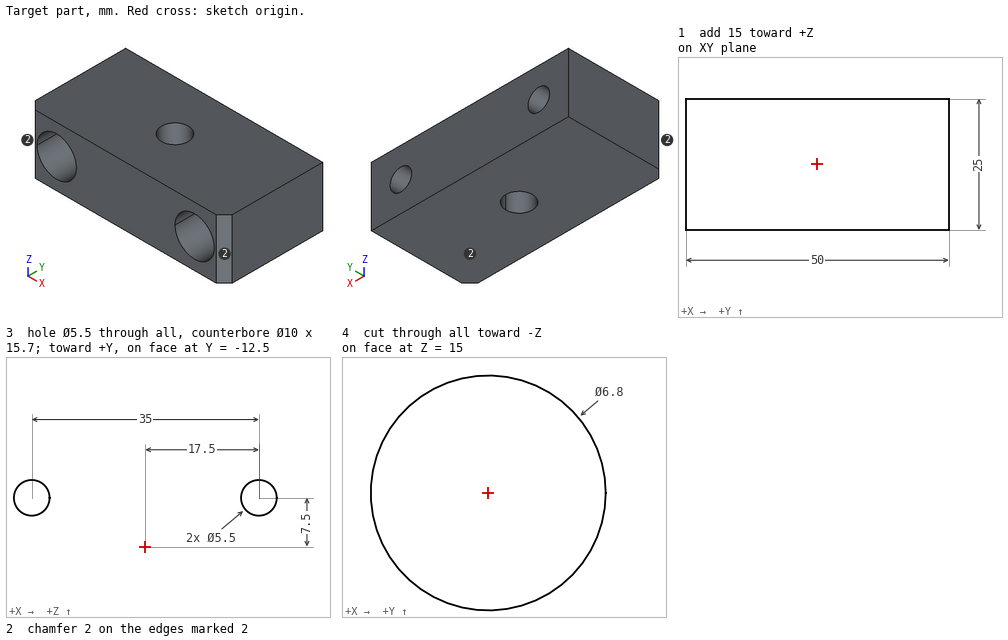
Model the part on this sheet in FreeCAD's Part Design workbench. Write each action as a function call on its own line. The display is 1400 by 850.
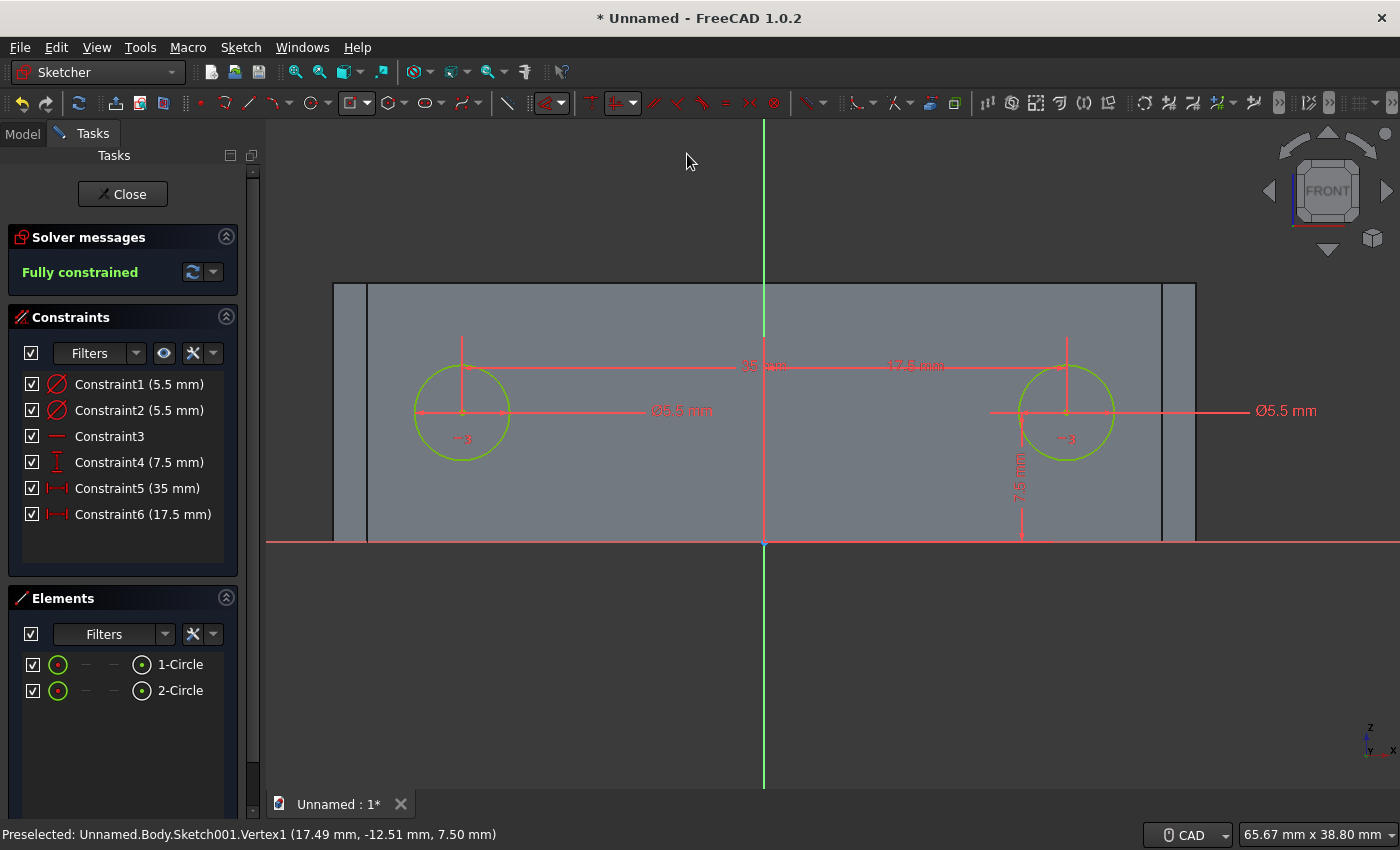
click(123, 194)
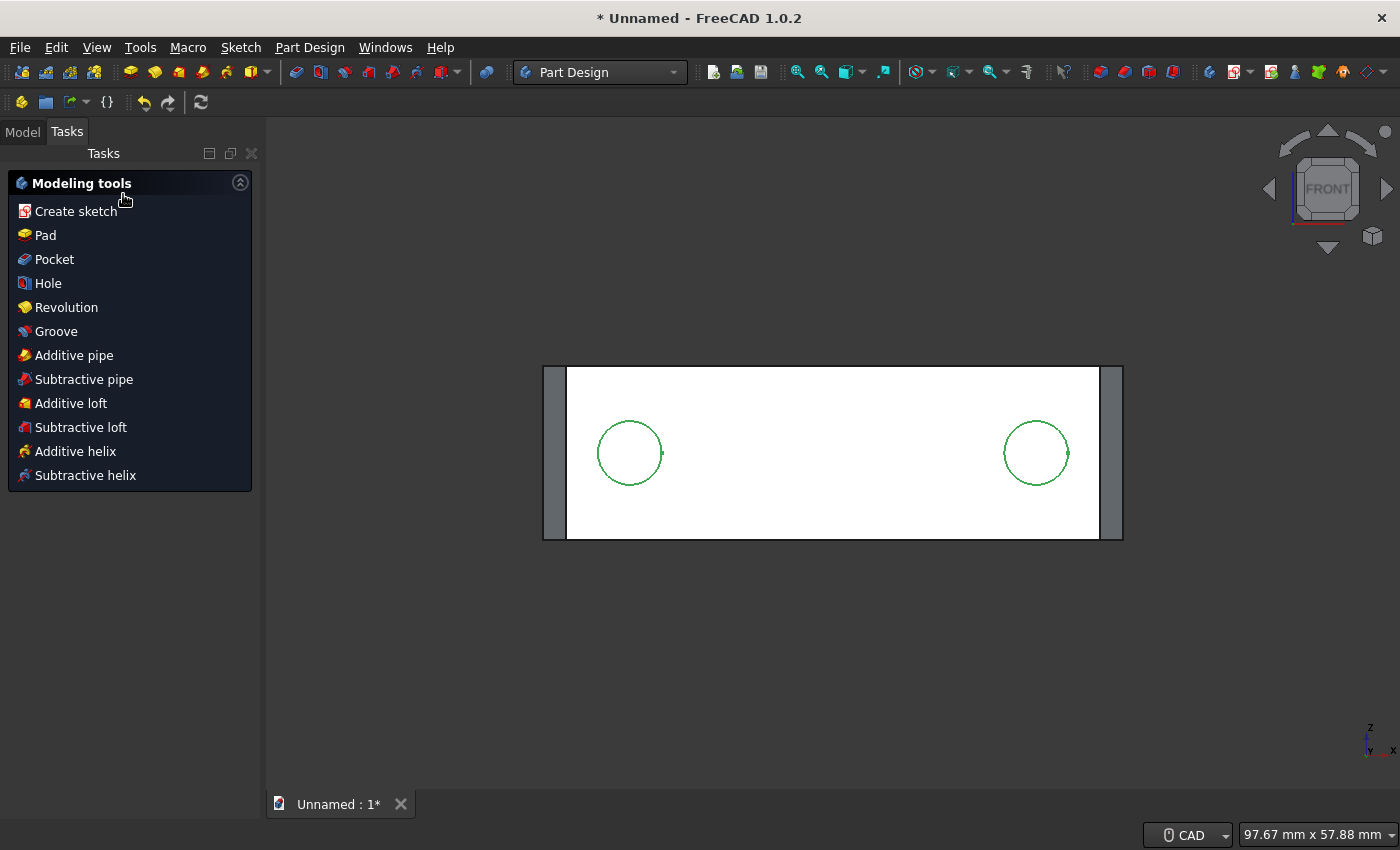
click(322, 72)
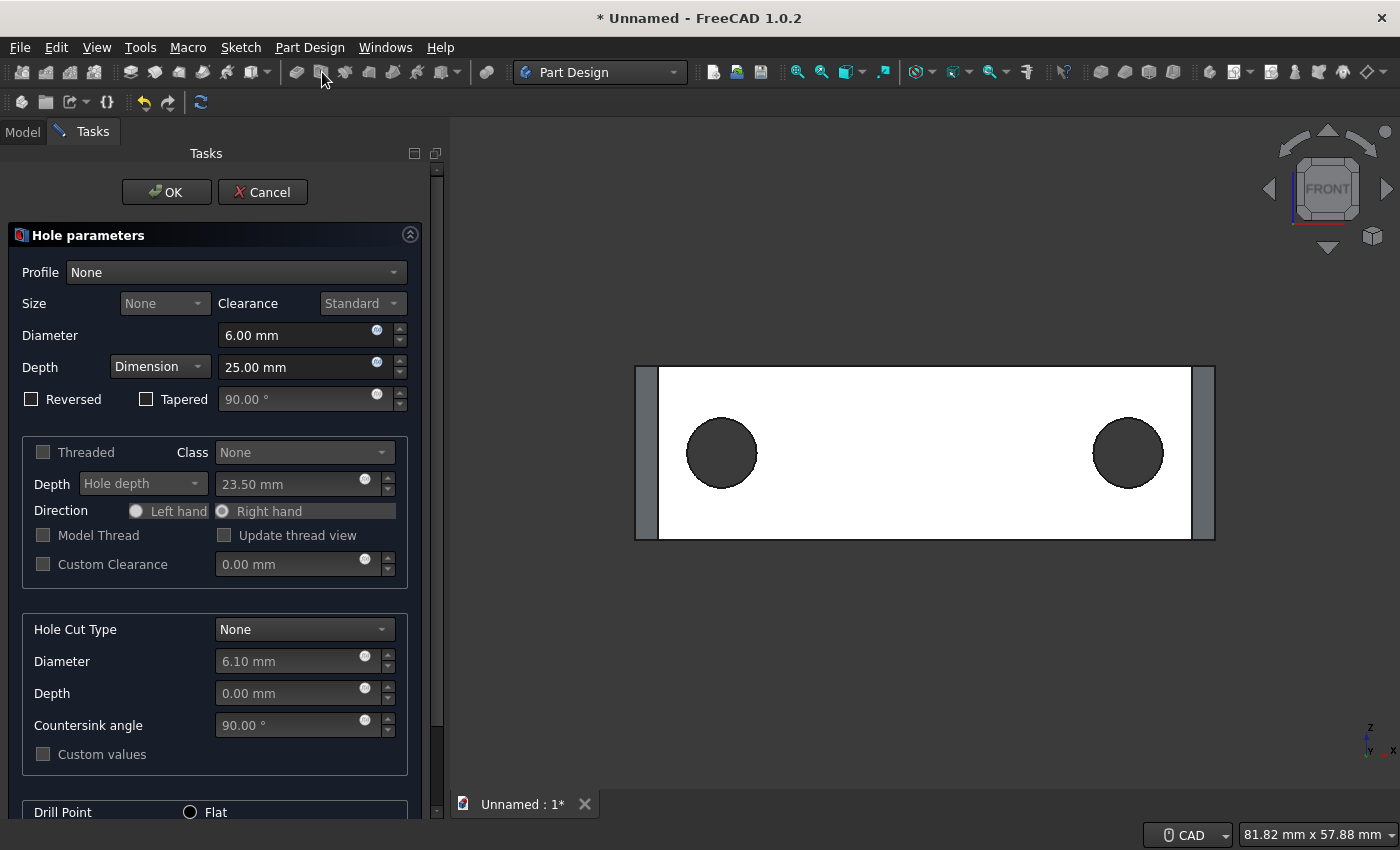
triple_click(305, 335)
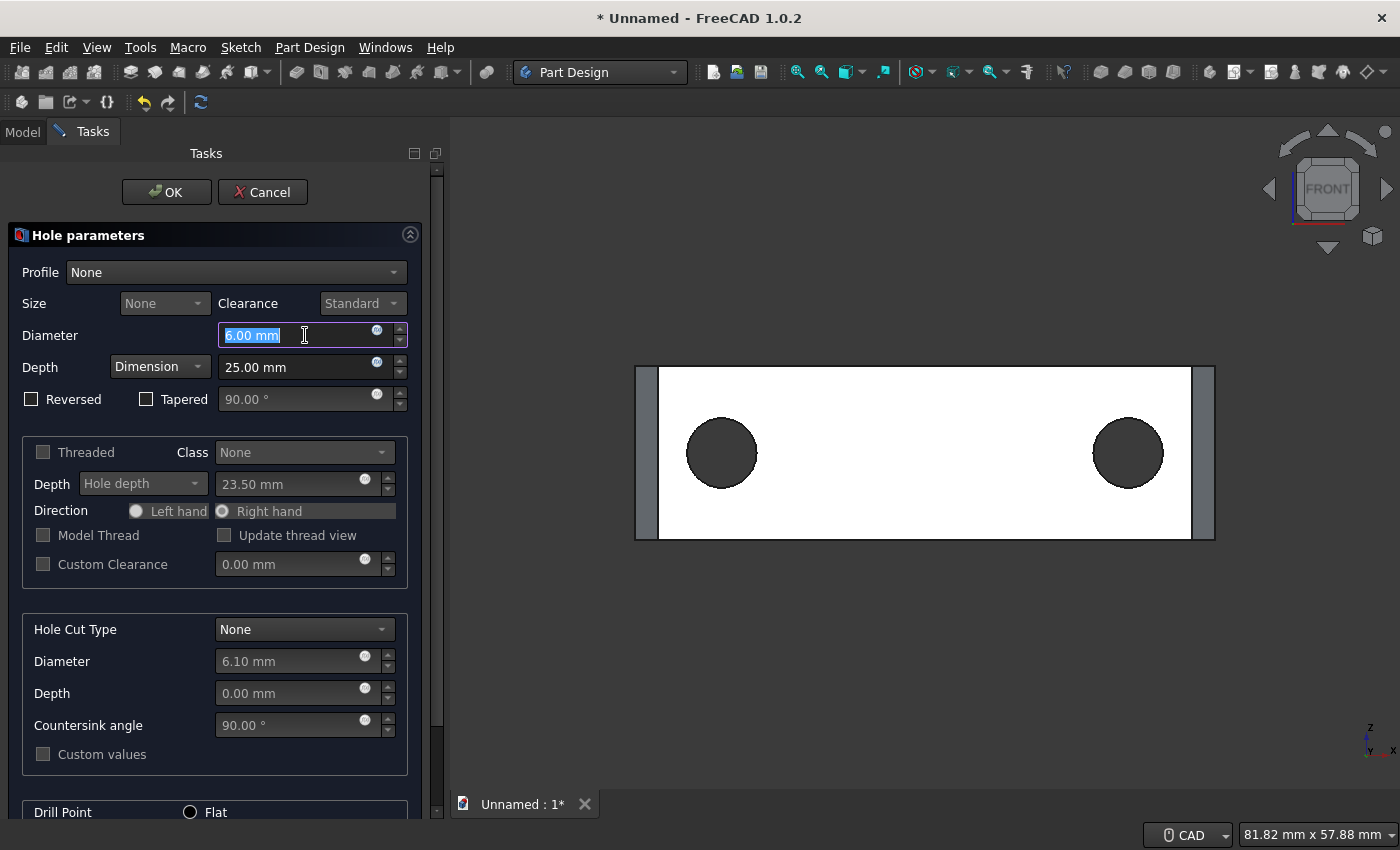
text(5.5)
key(Tab)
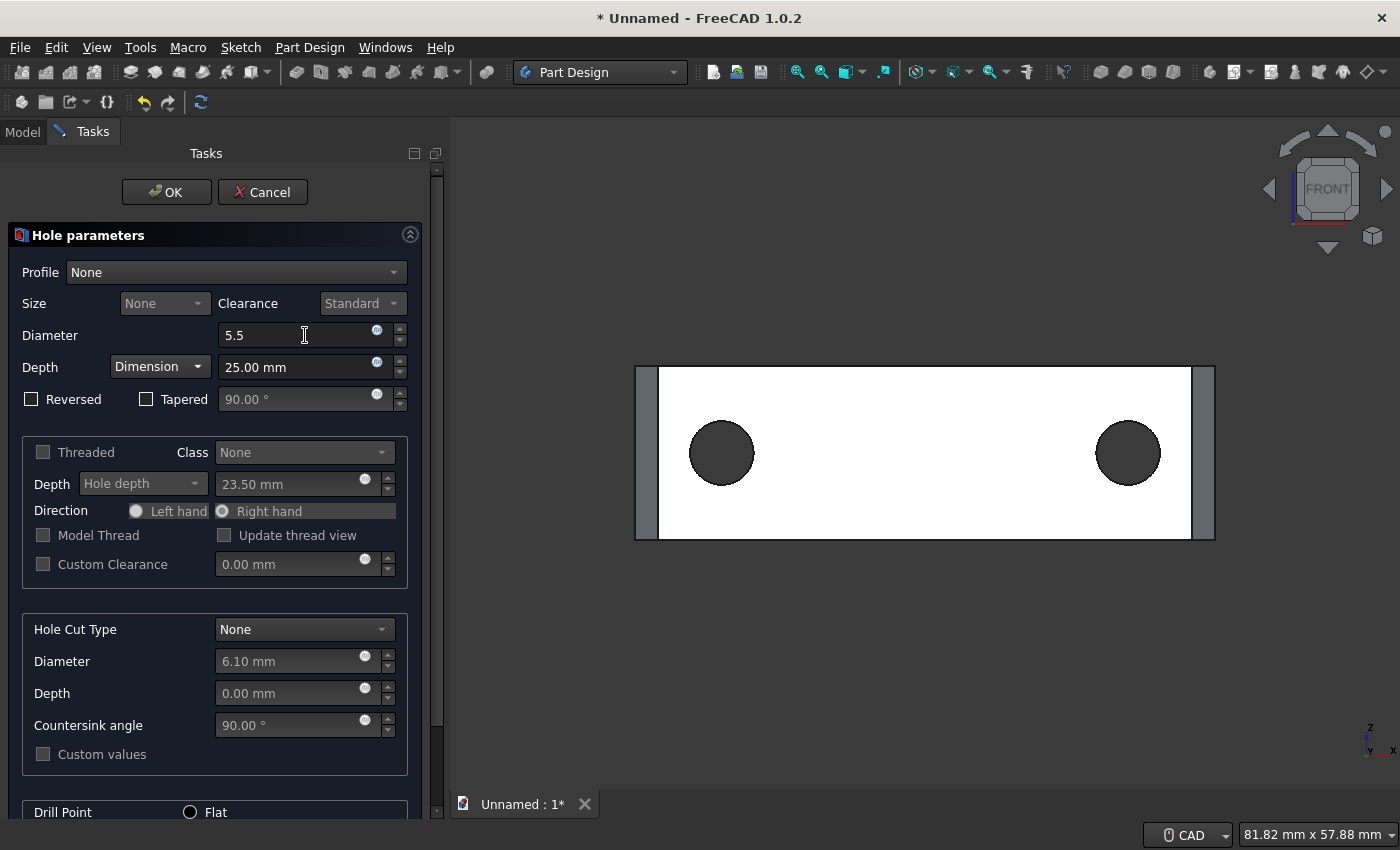
click(161, 366)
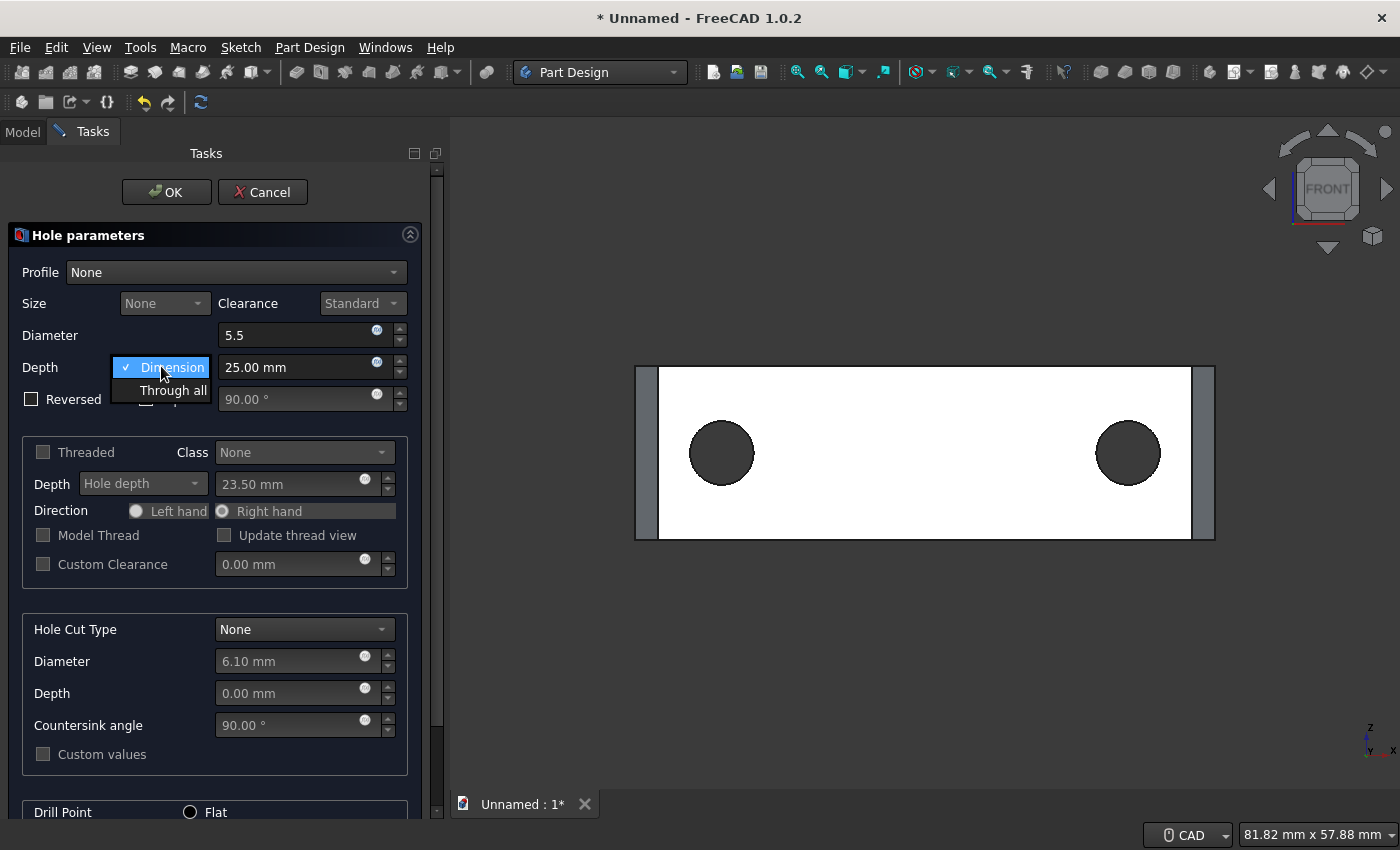
click(160, 390)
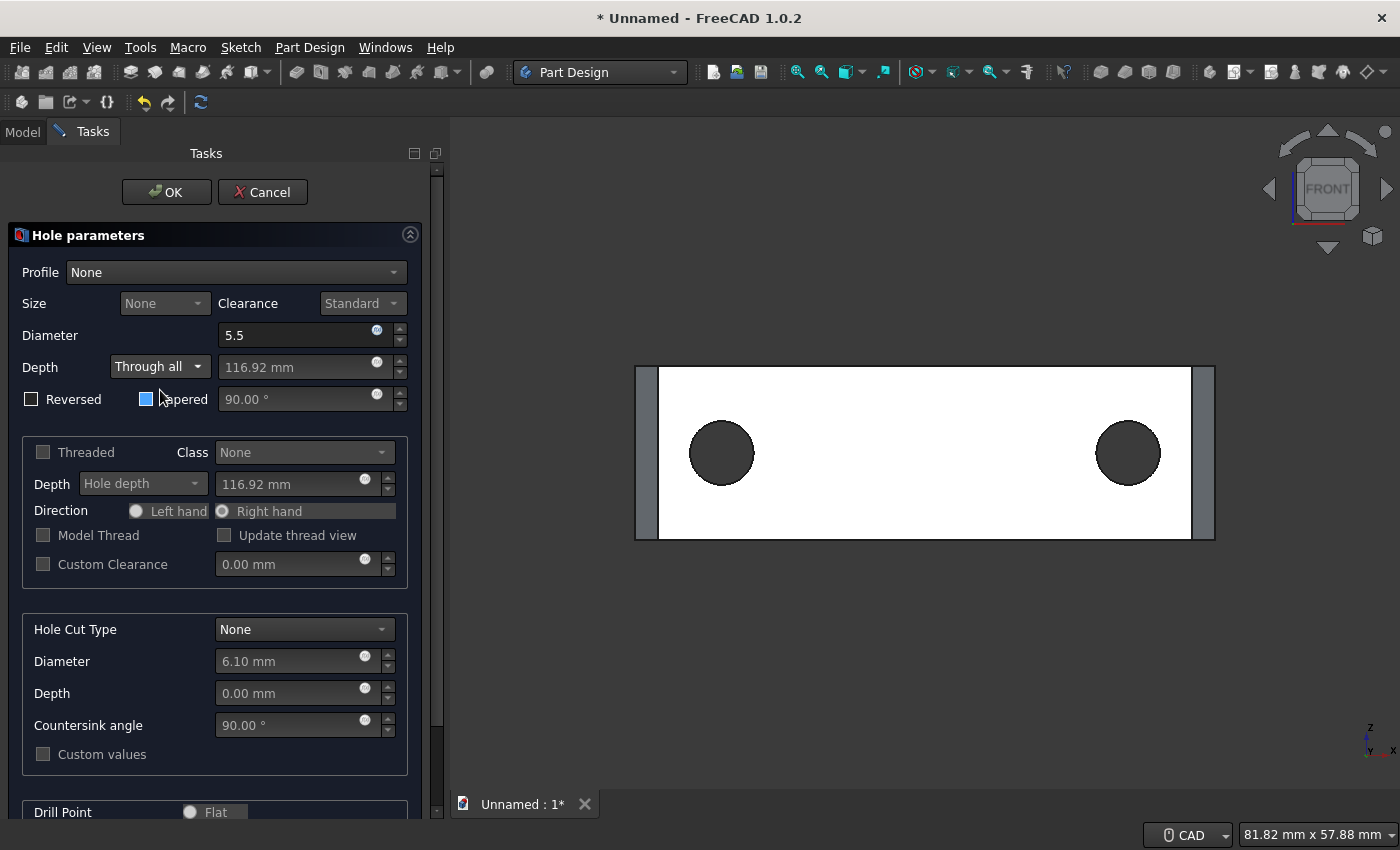
click(306, 630)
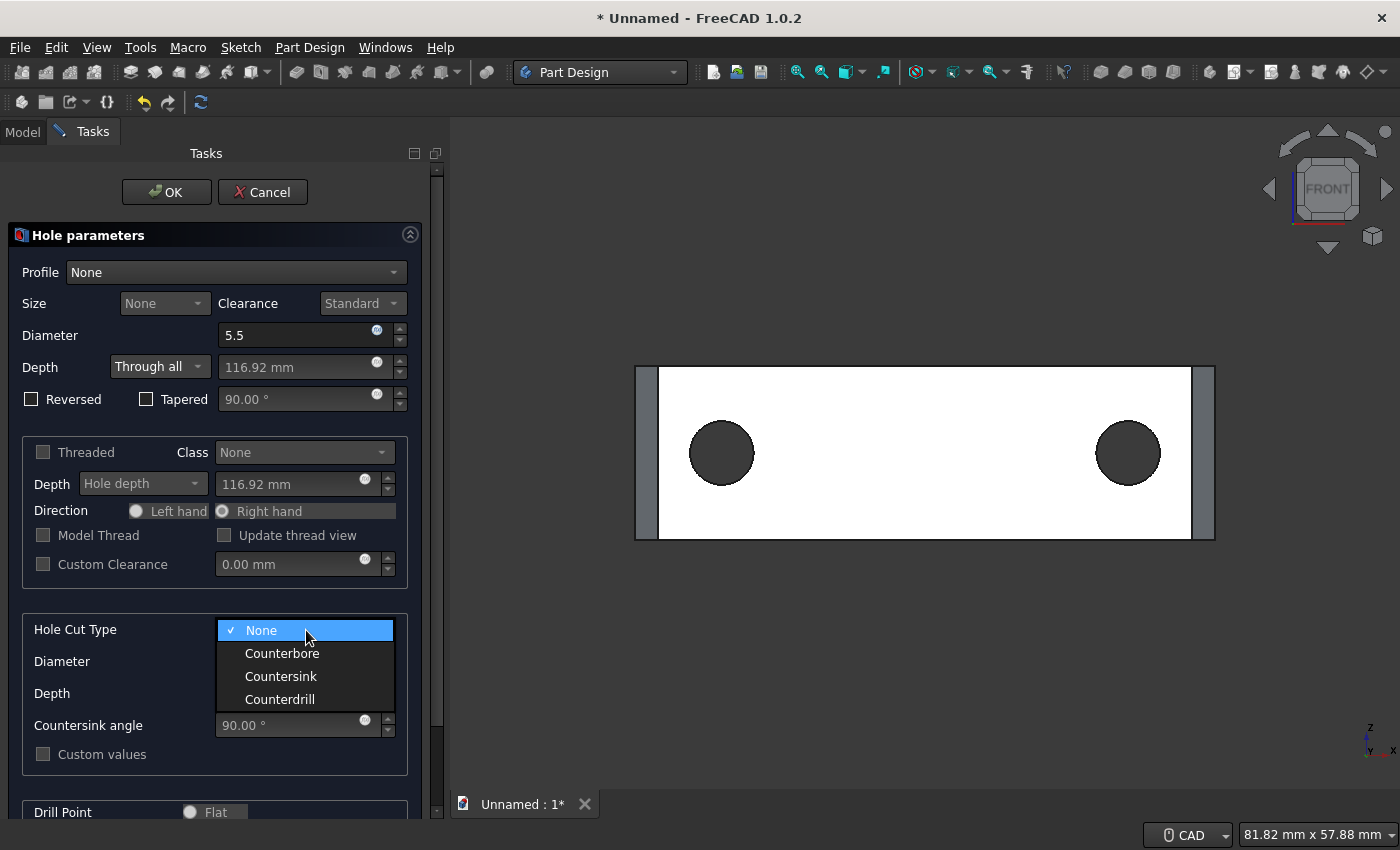
click(304, 654)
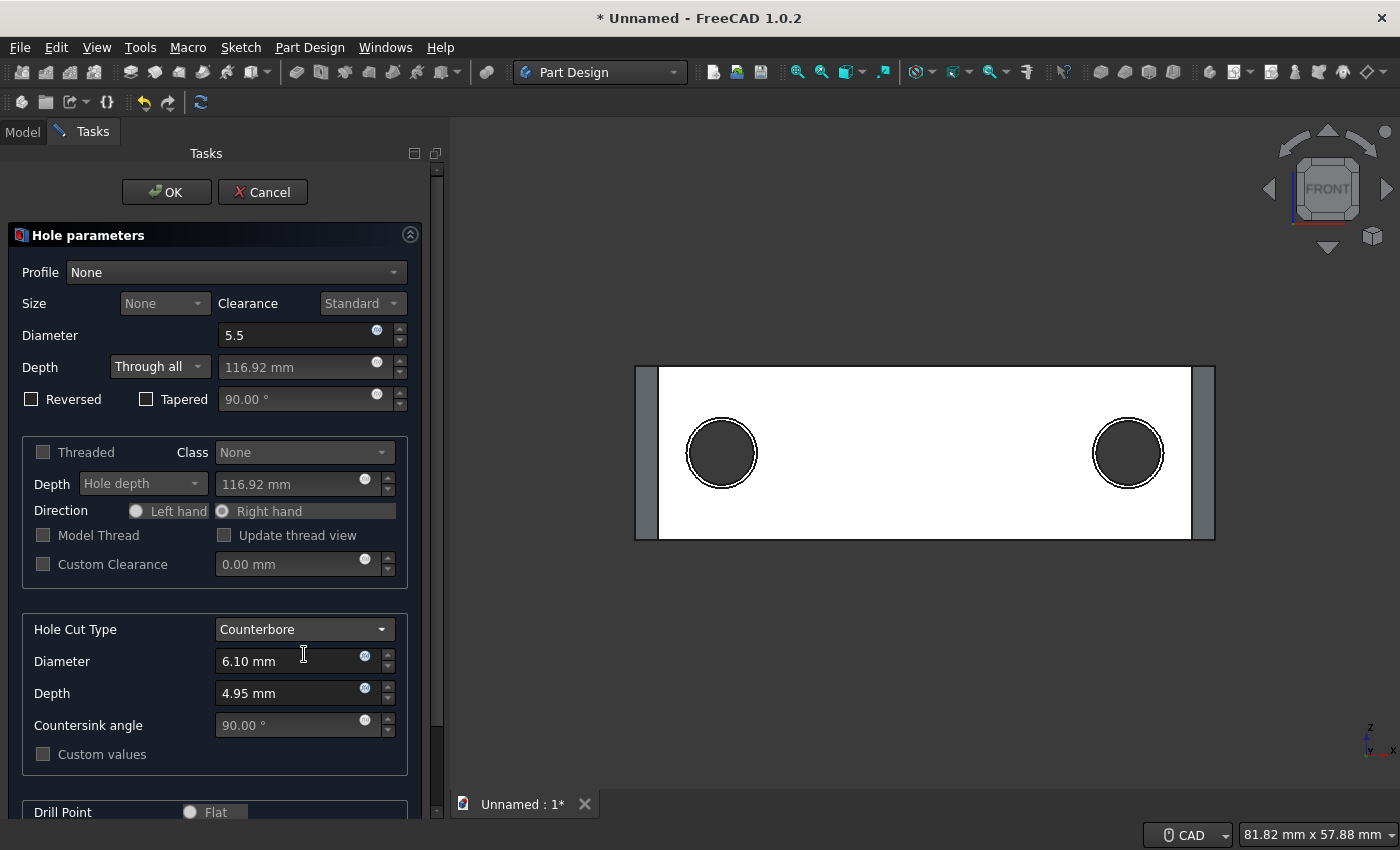
triple_click(298, 661)